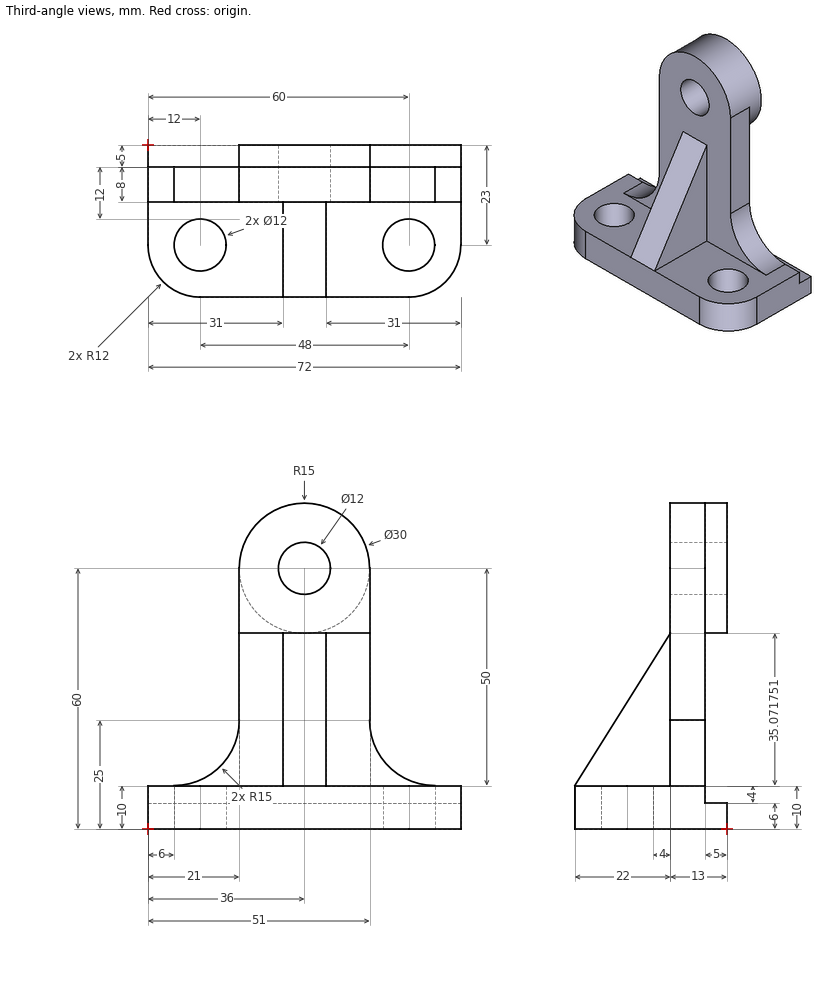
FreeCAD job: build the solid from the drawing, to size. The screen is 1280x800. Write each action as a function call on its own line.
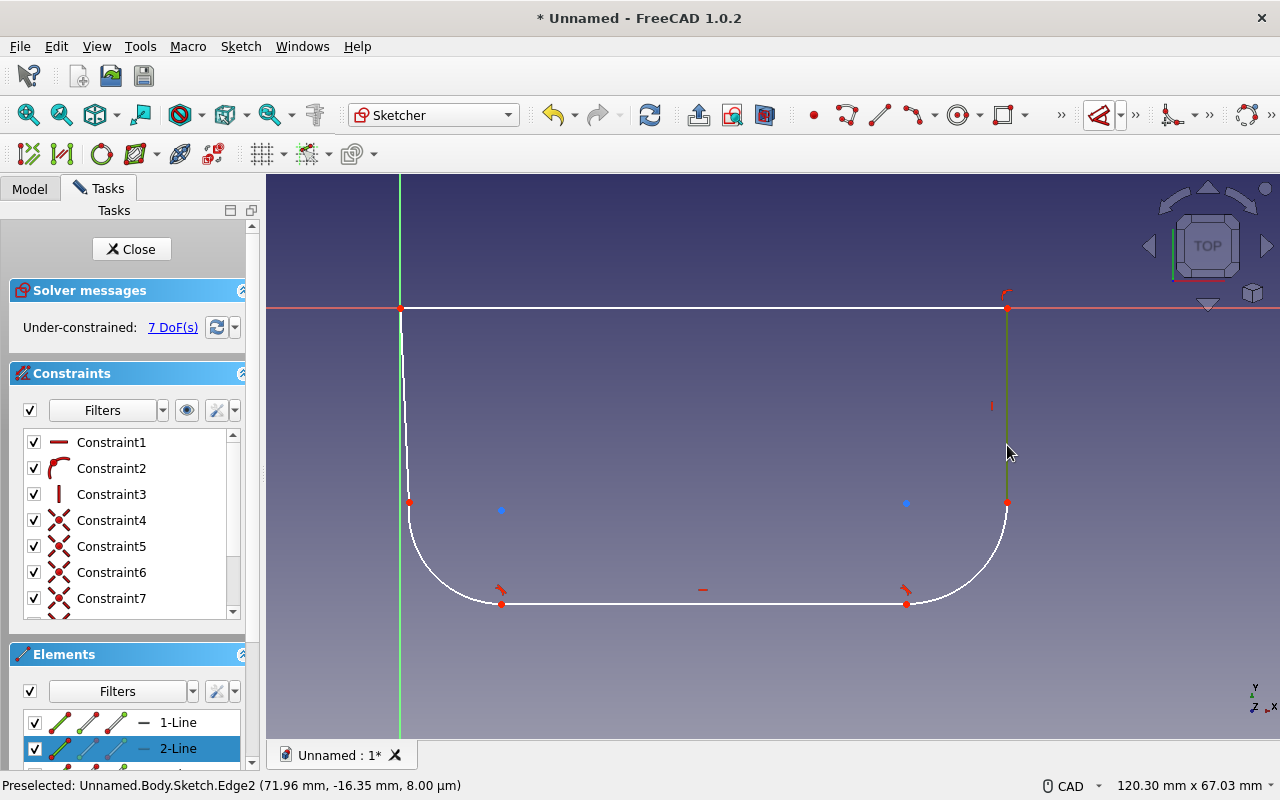
click(952, 593)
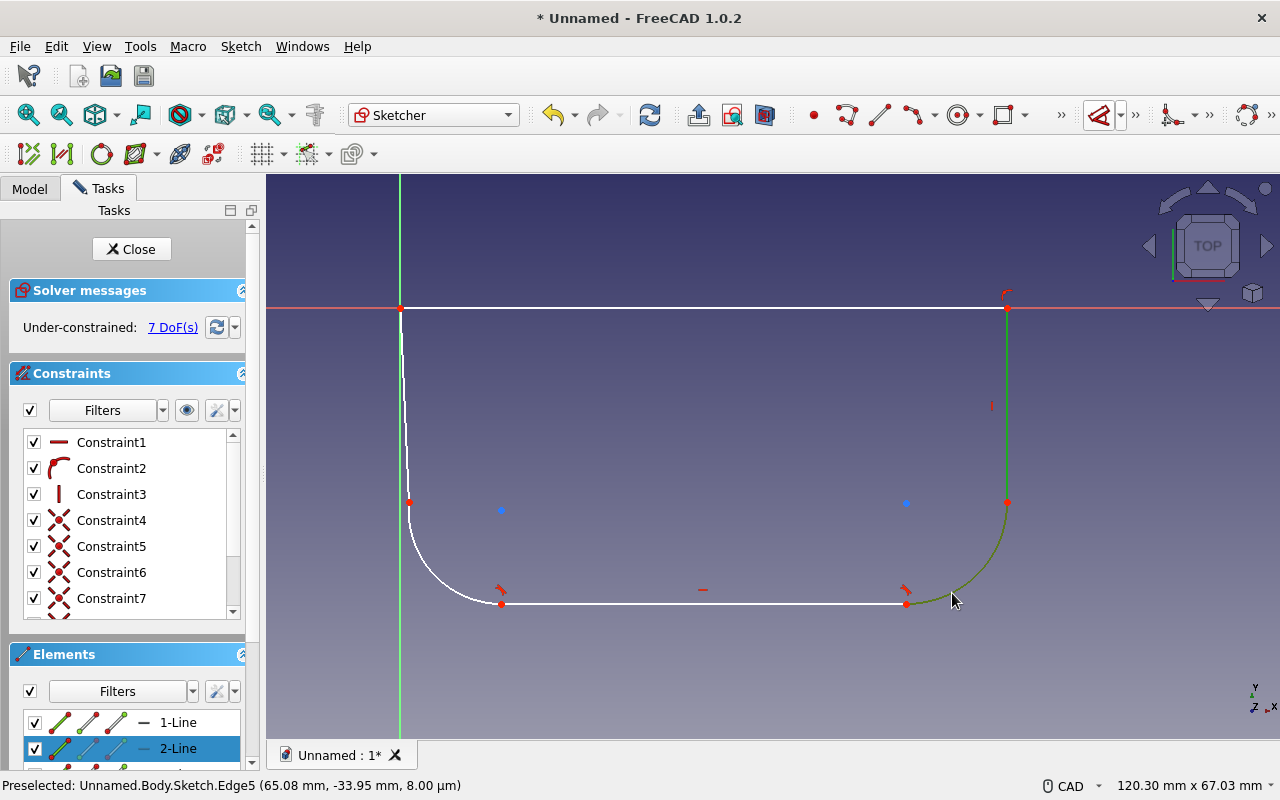
key(t)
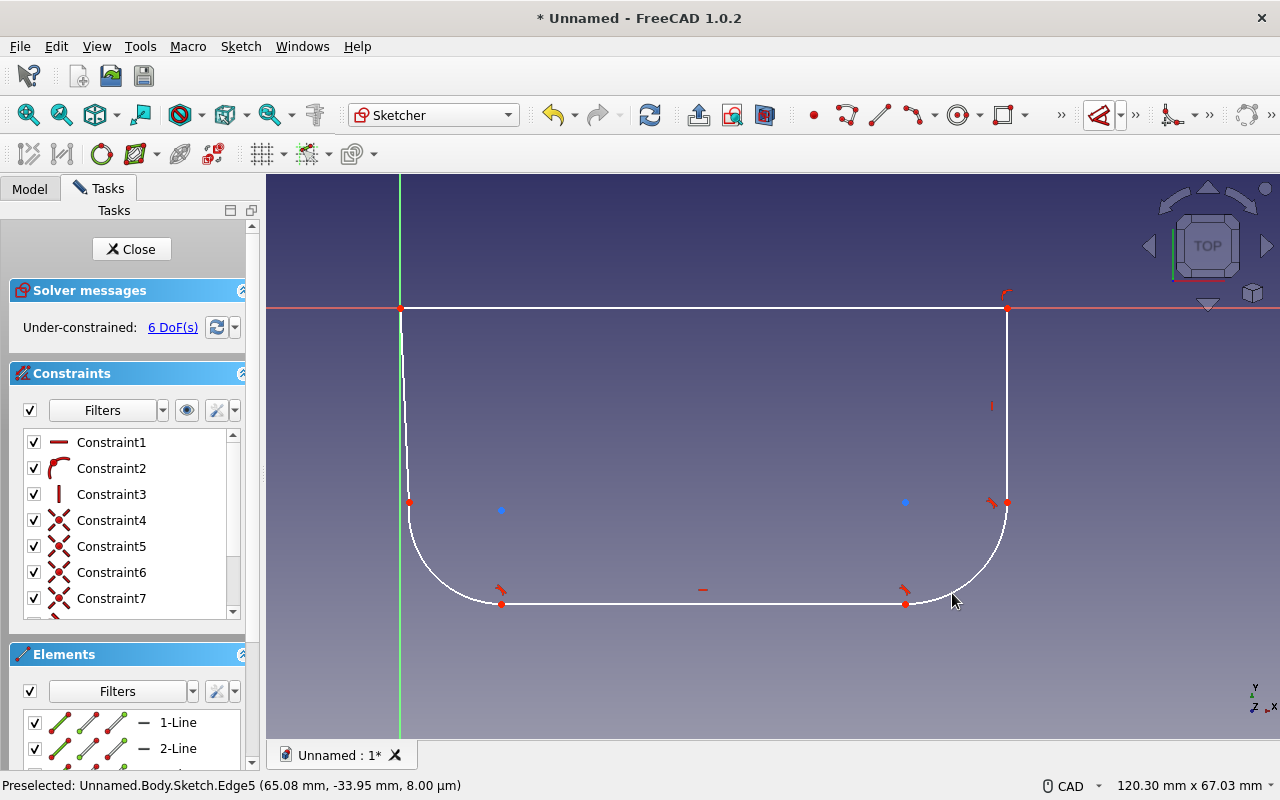
click(403, 367)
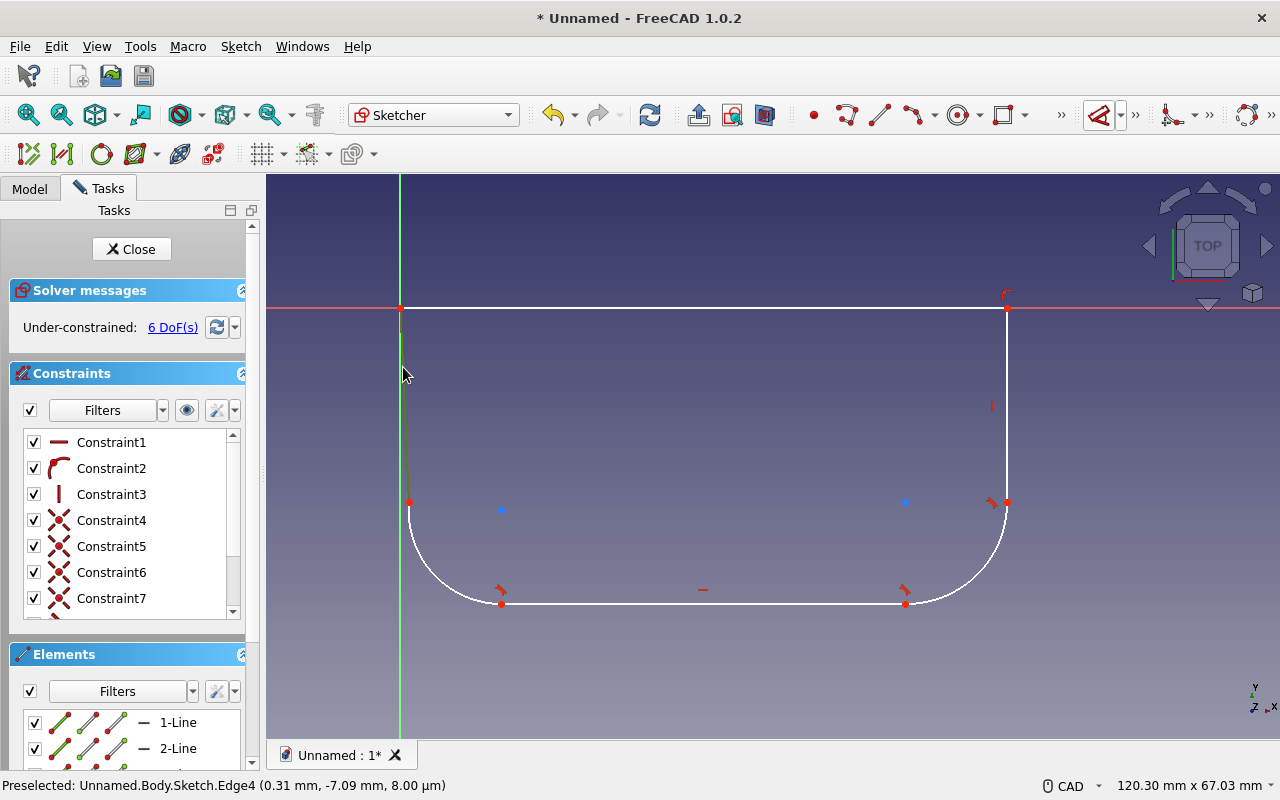
click(417, 548)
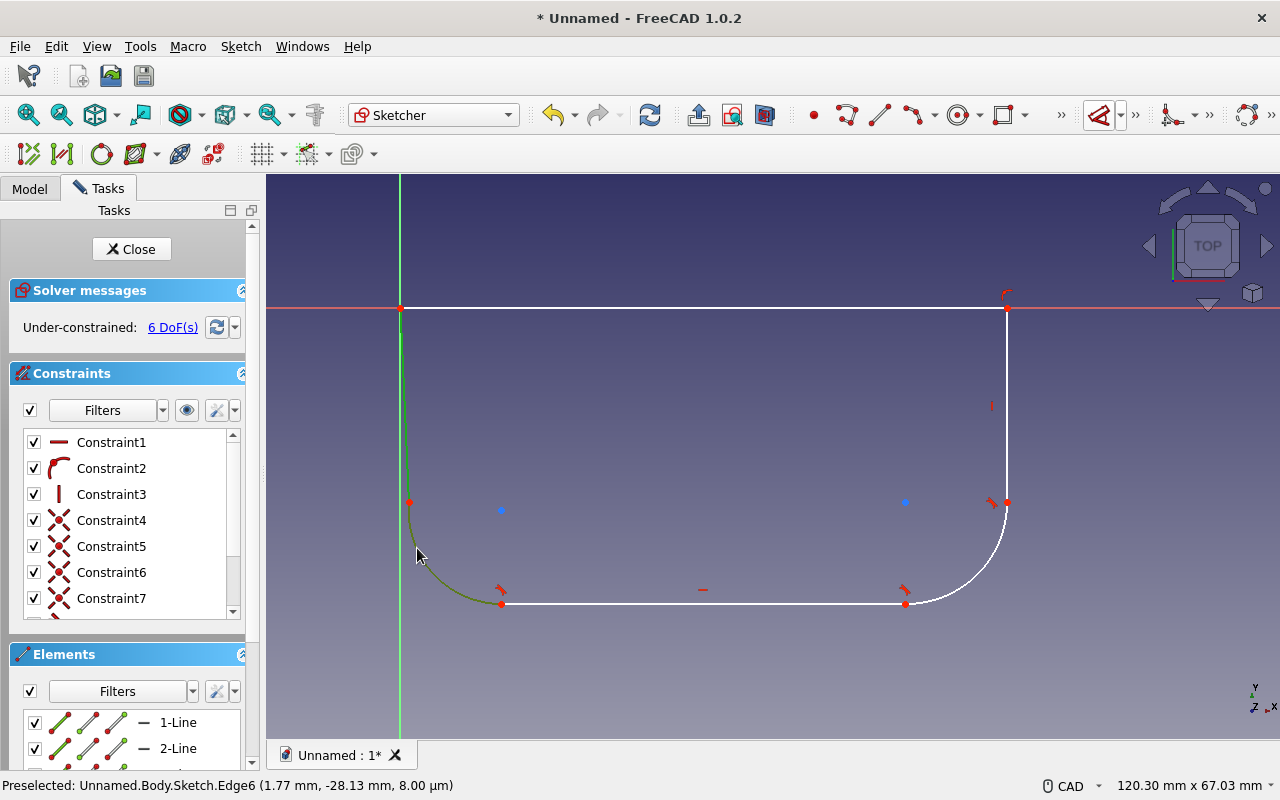
key(t)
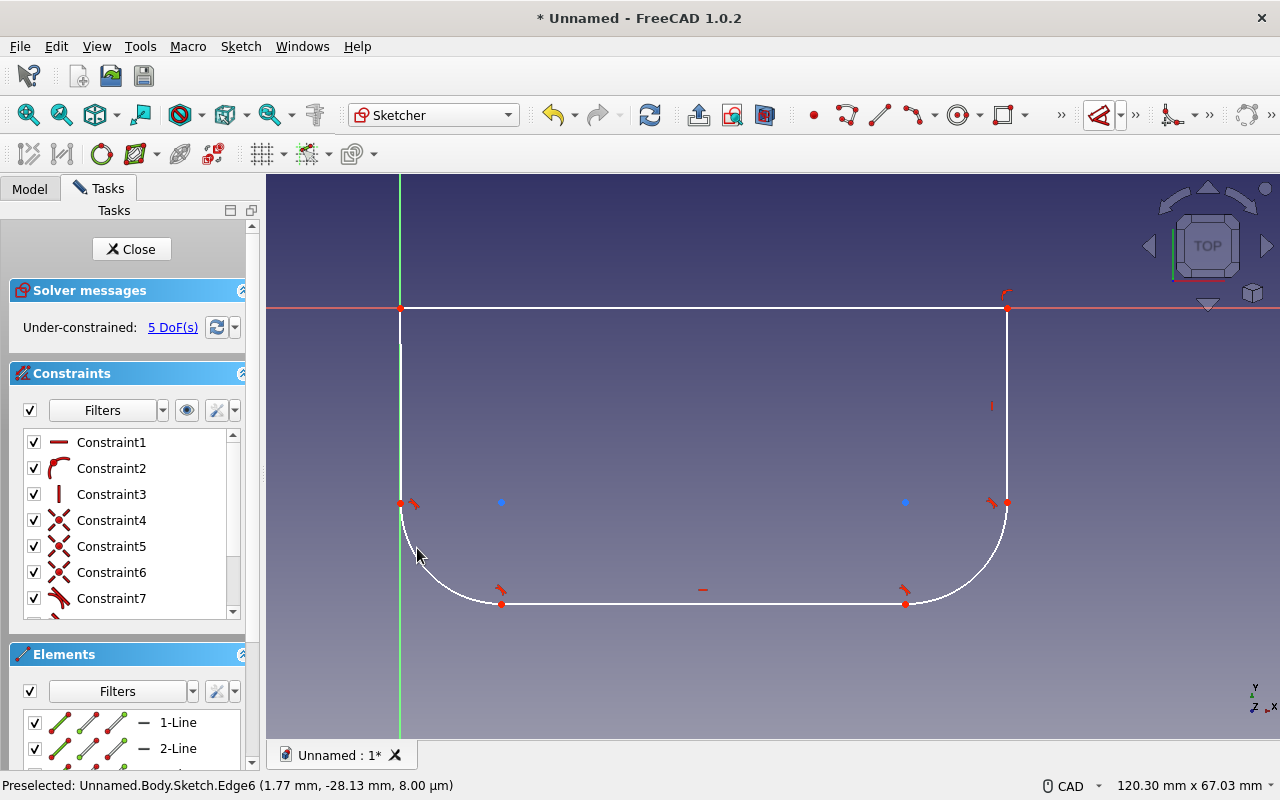
click(401, 367)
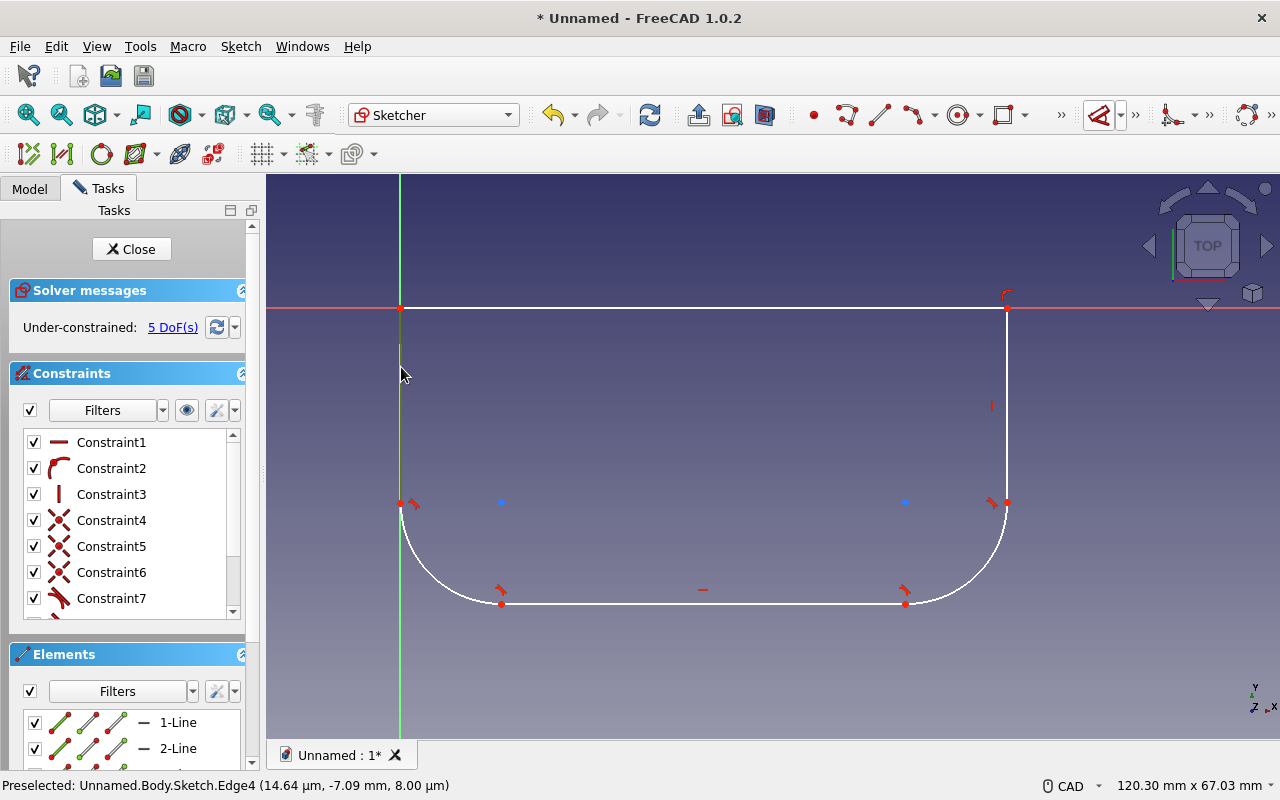
key(v)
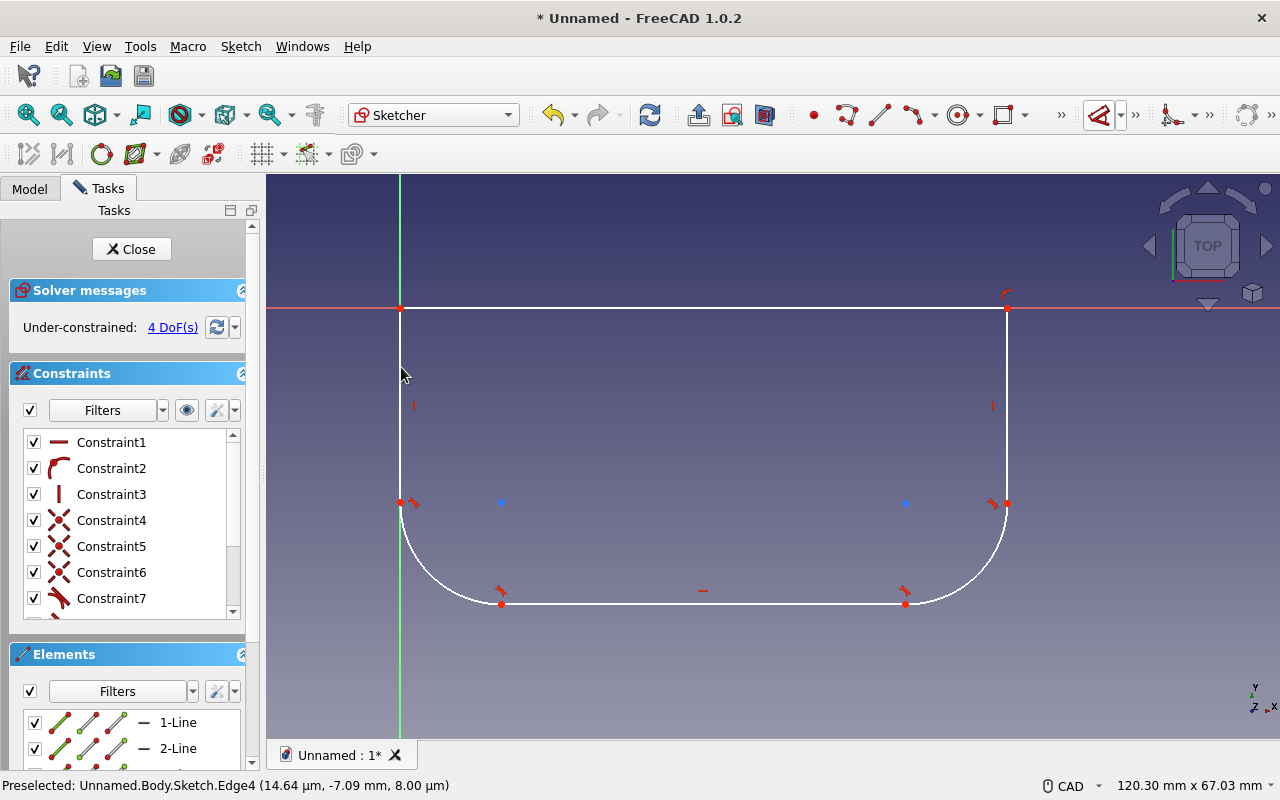
click(952, 593)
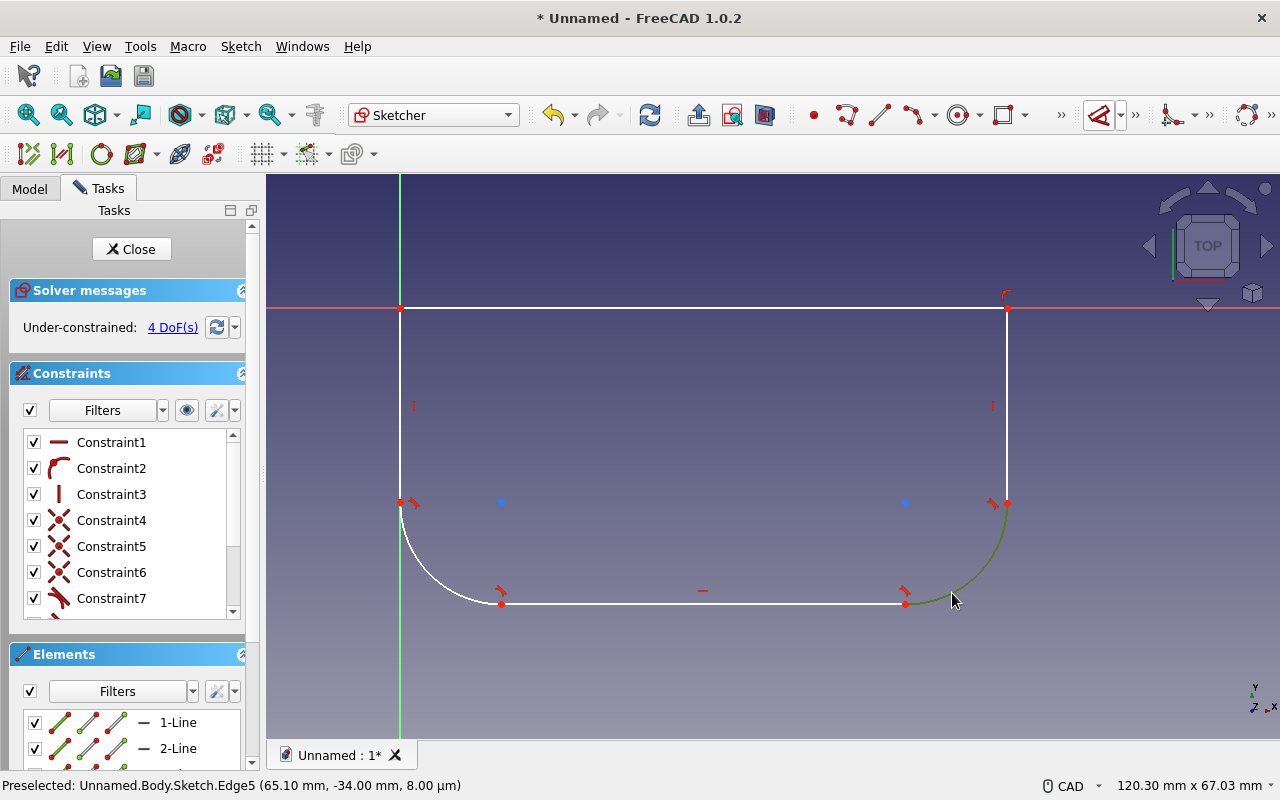
scroll(411, 549, up, 2)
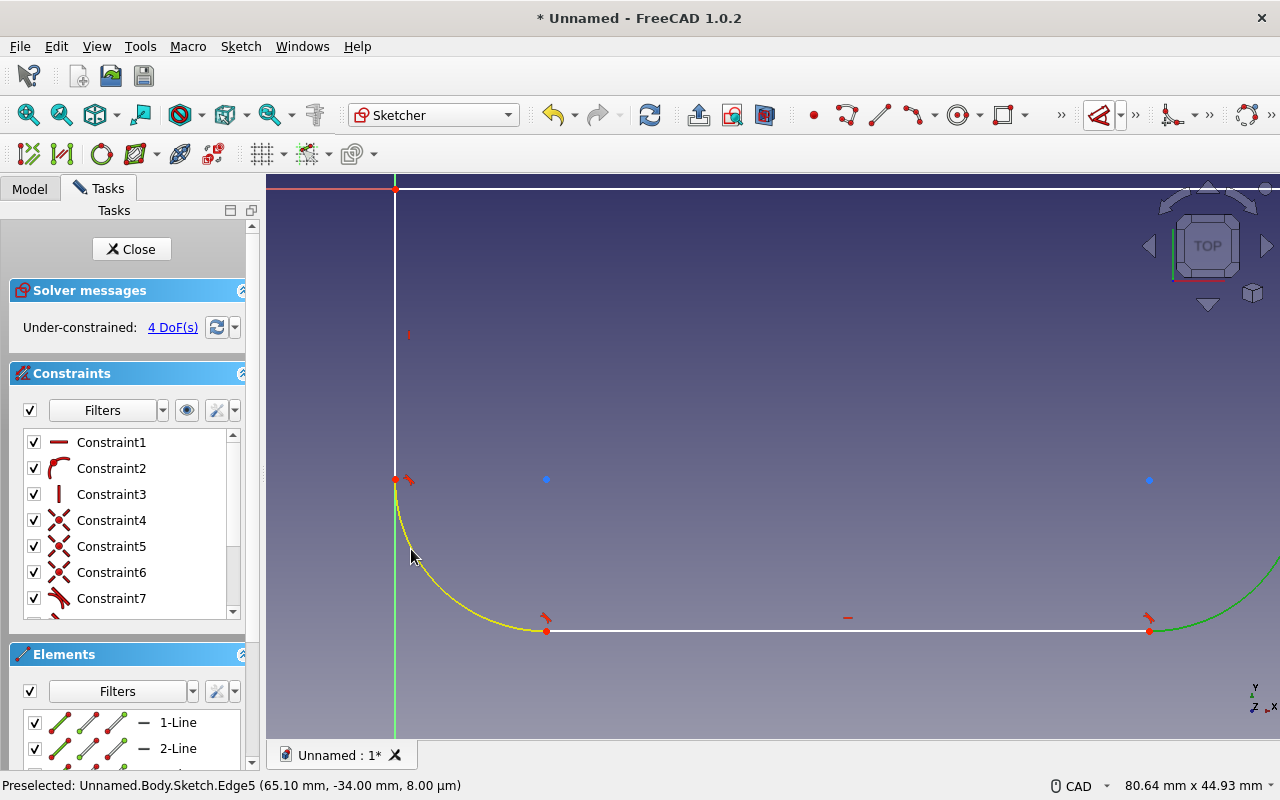
click(412, 549)